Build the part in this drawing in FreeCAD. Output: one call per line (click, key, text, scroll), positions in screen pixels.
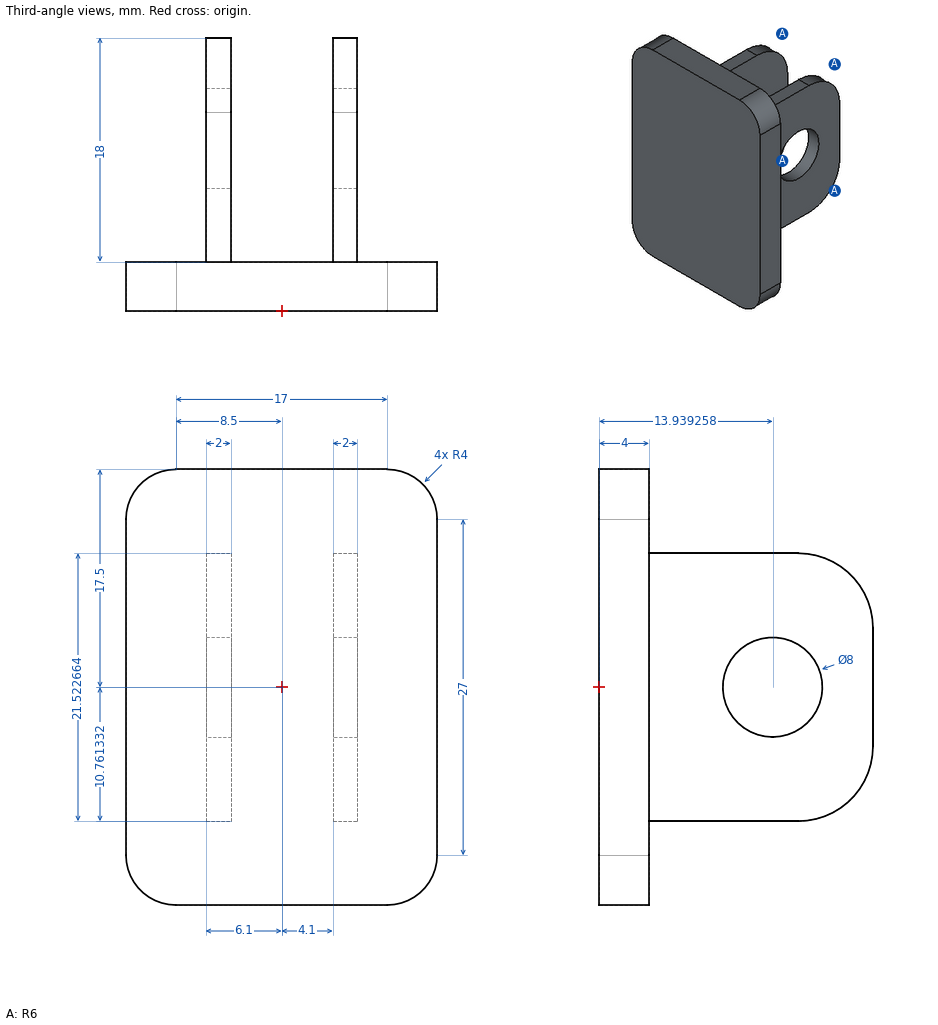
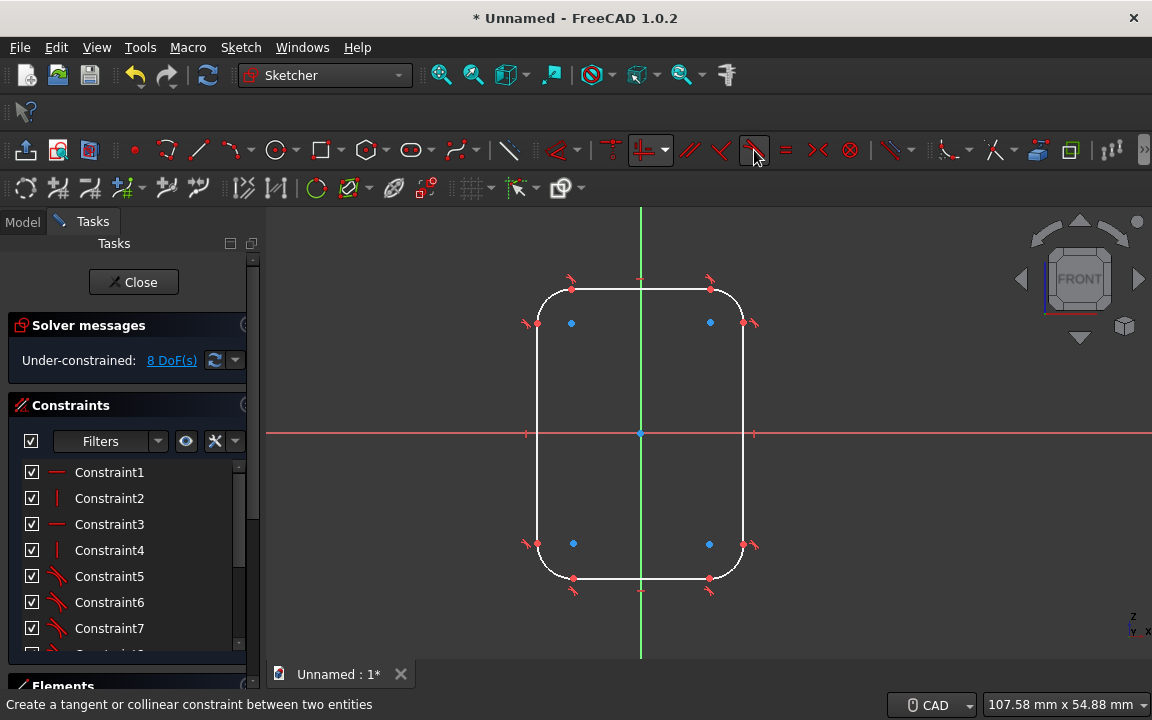
click(740, 307)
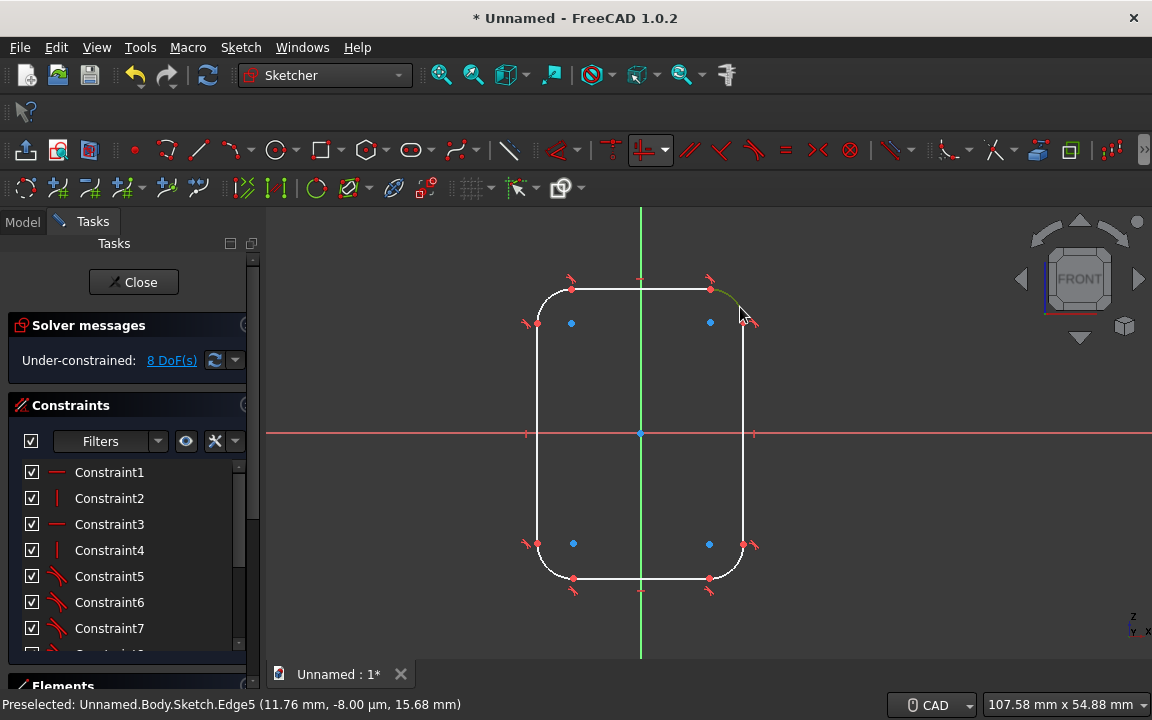
click(725, 575)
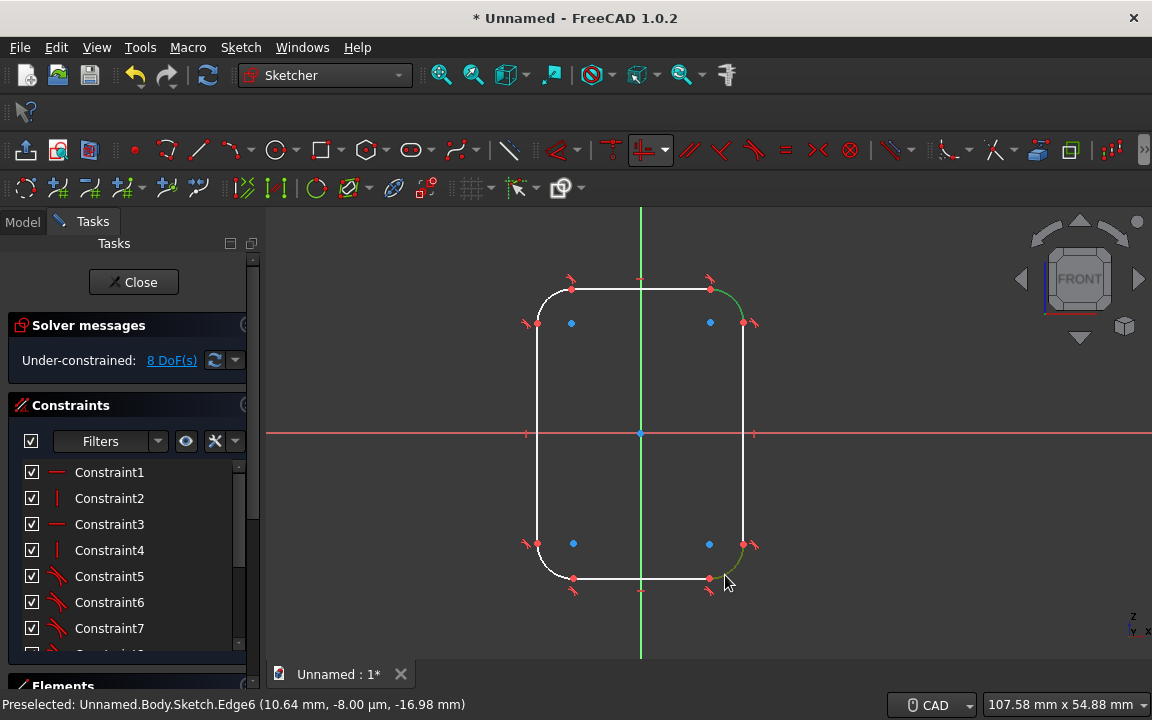
click(541, 559)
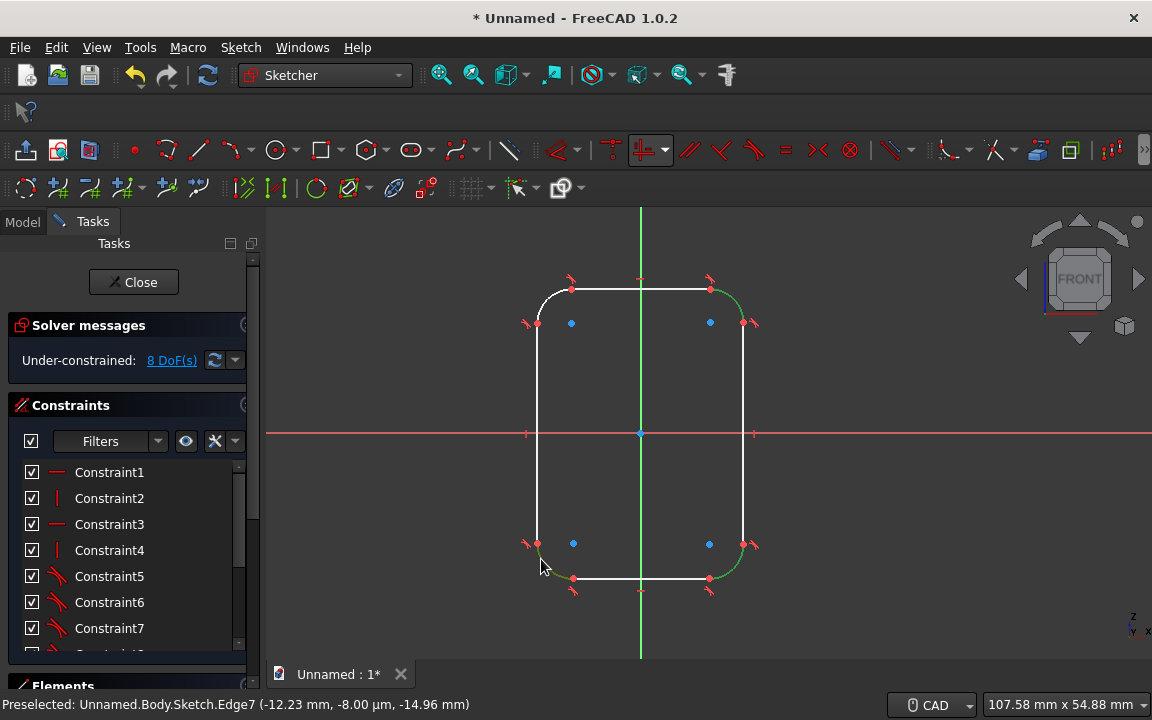
click(556, 293)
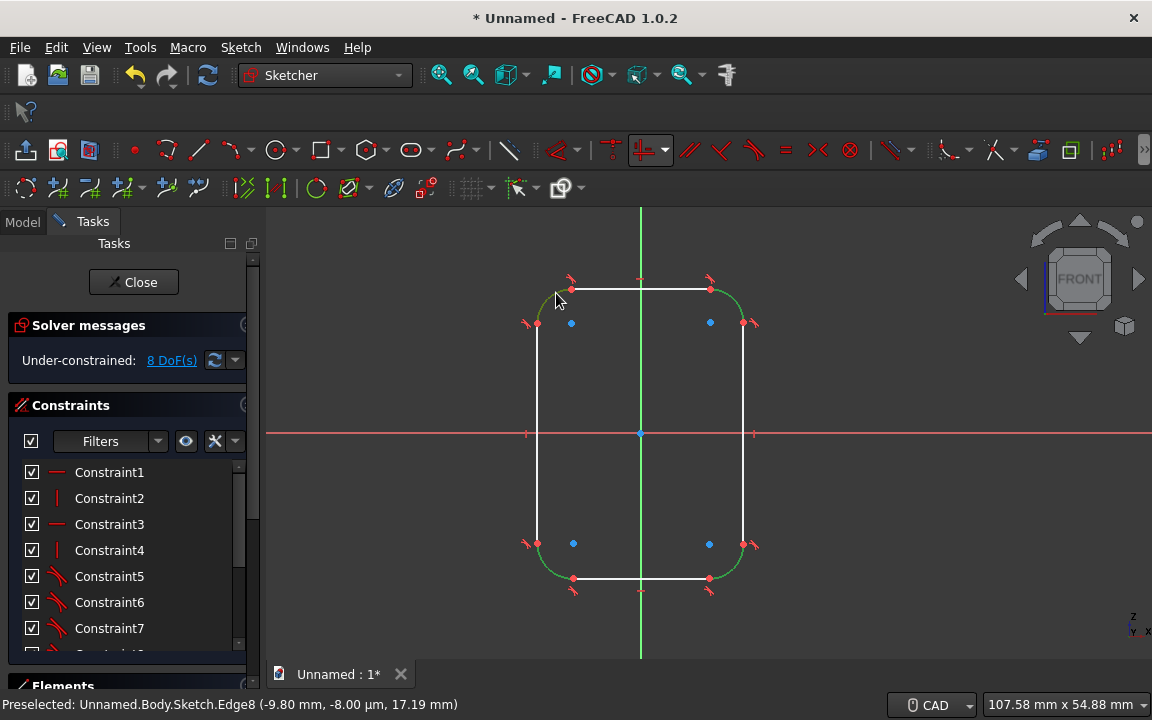
click(786, 150)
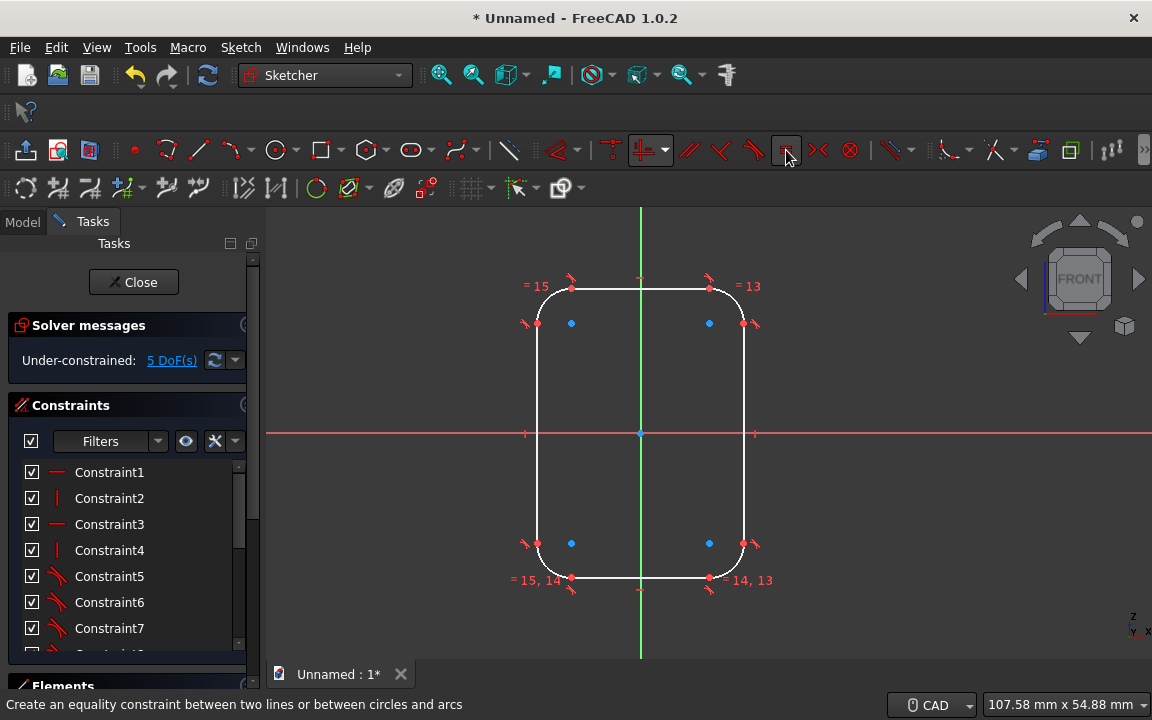
click(556, 150)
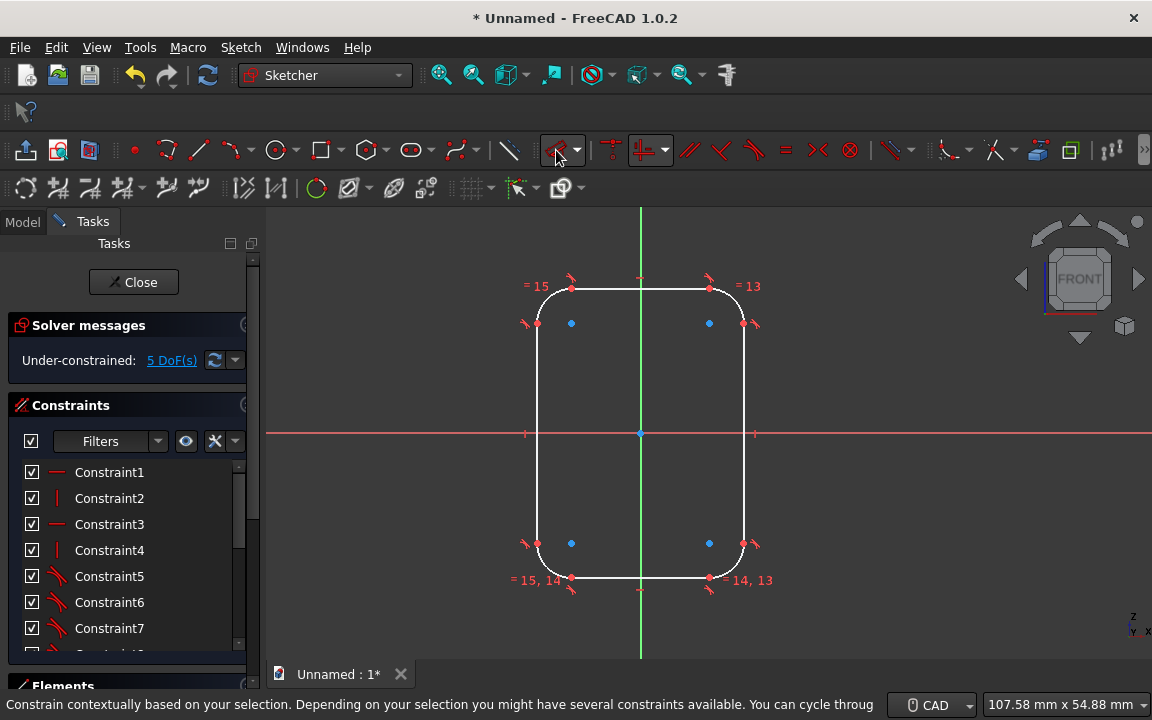
click(740, 308)
click(769, 293)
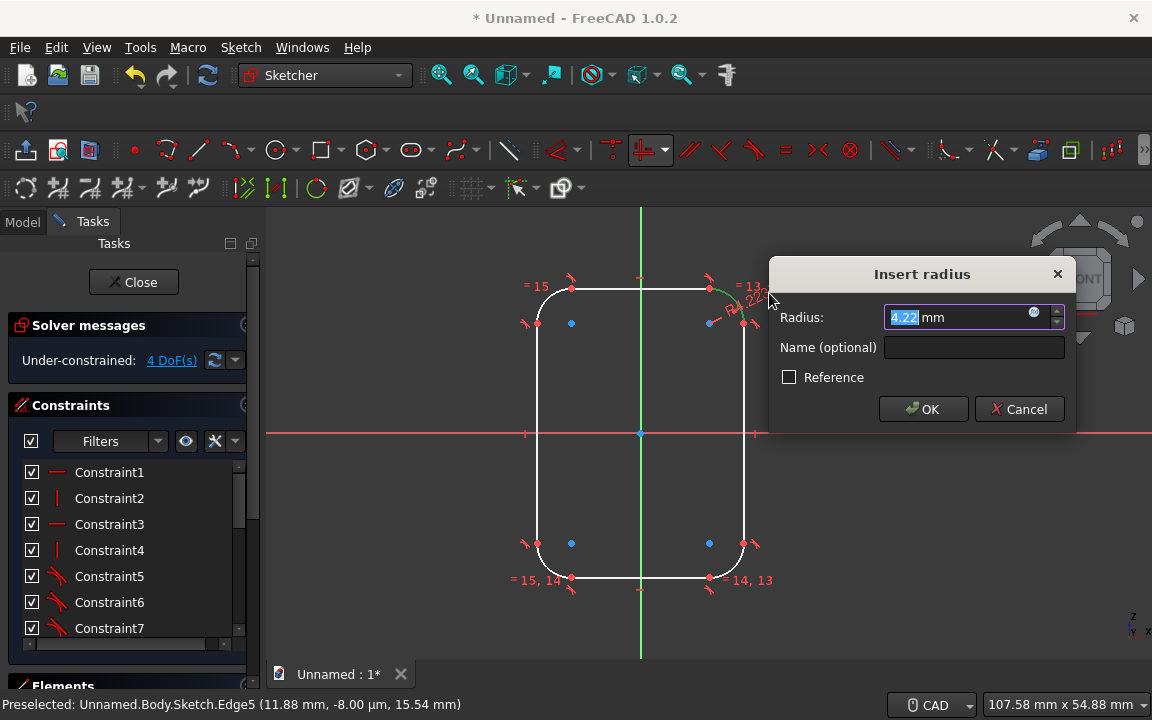
text(4)
key(Return)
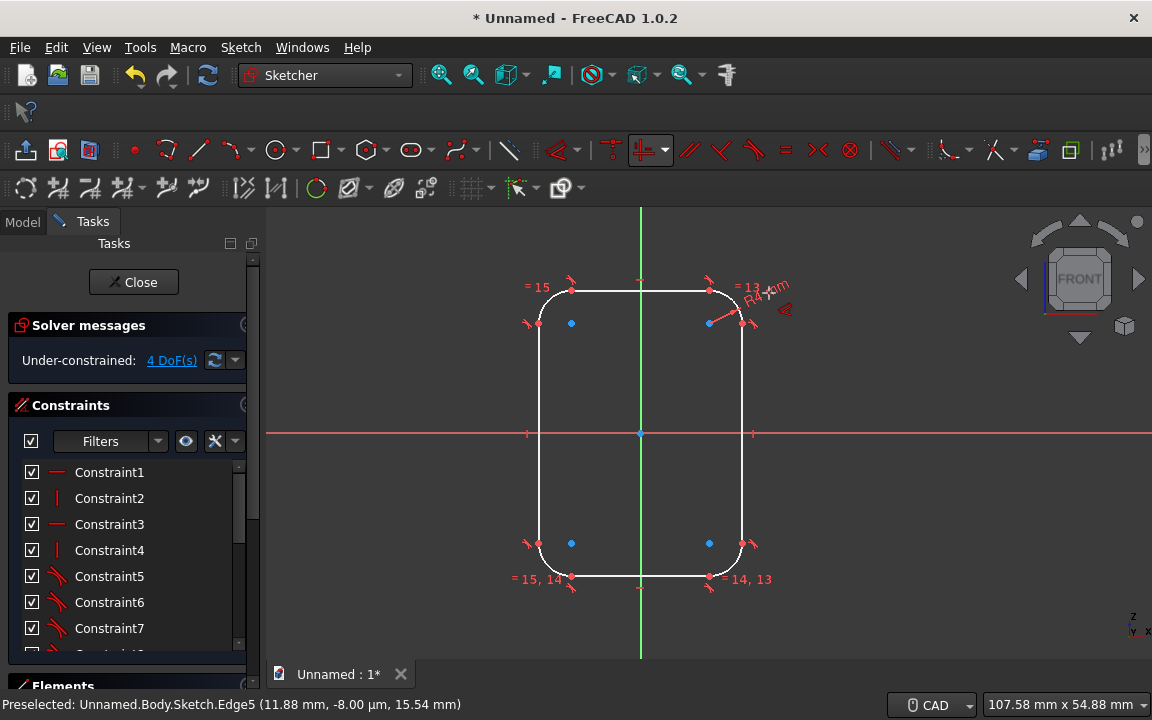
click(613, 291)
click(609, 257)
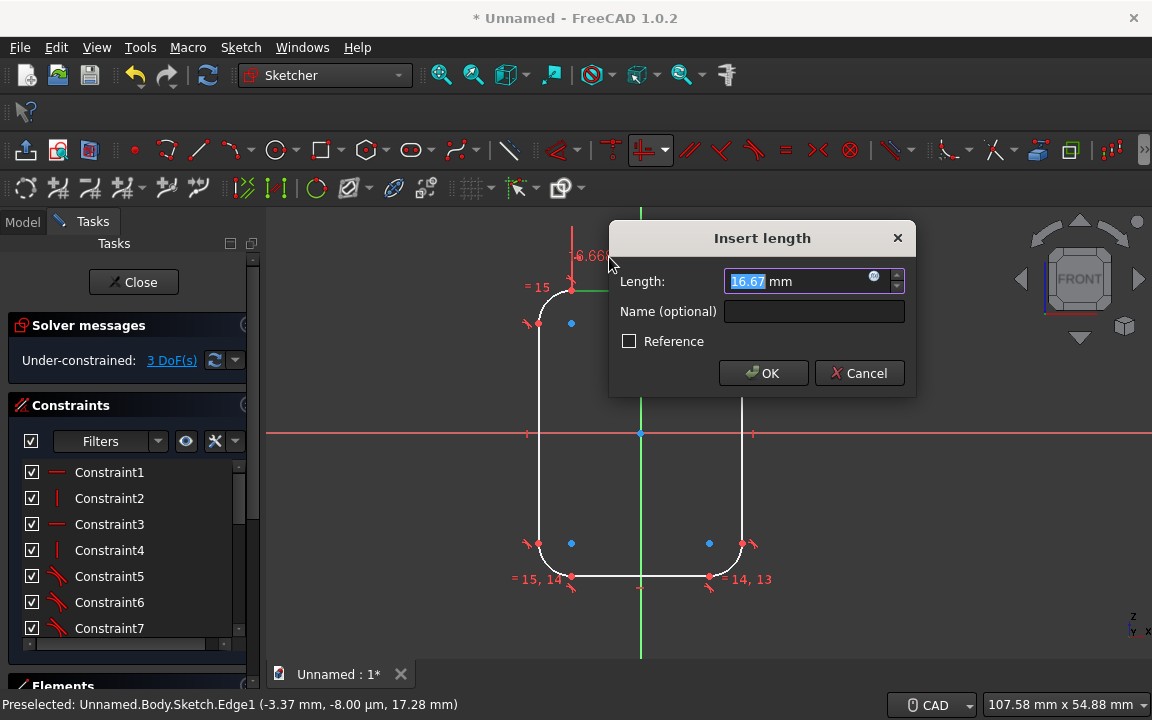
text(17)
key(Return)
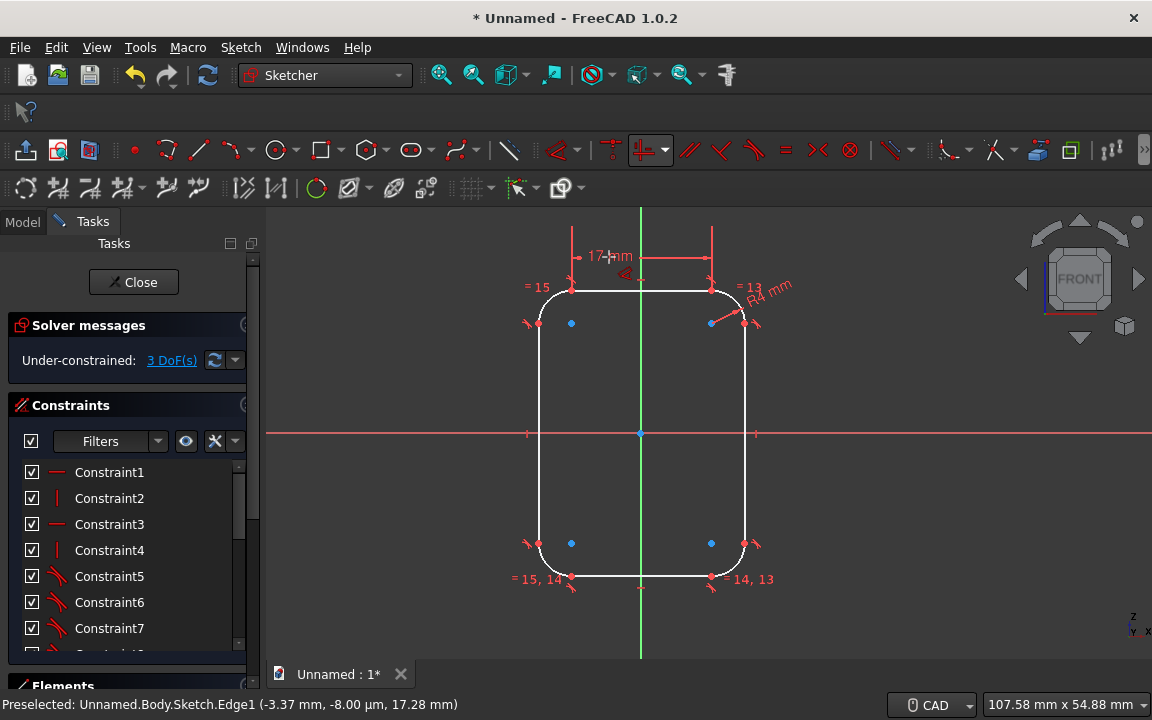
click(745, 390)
click(779, 383)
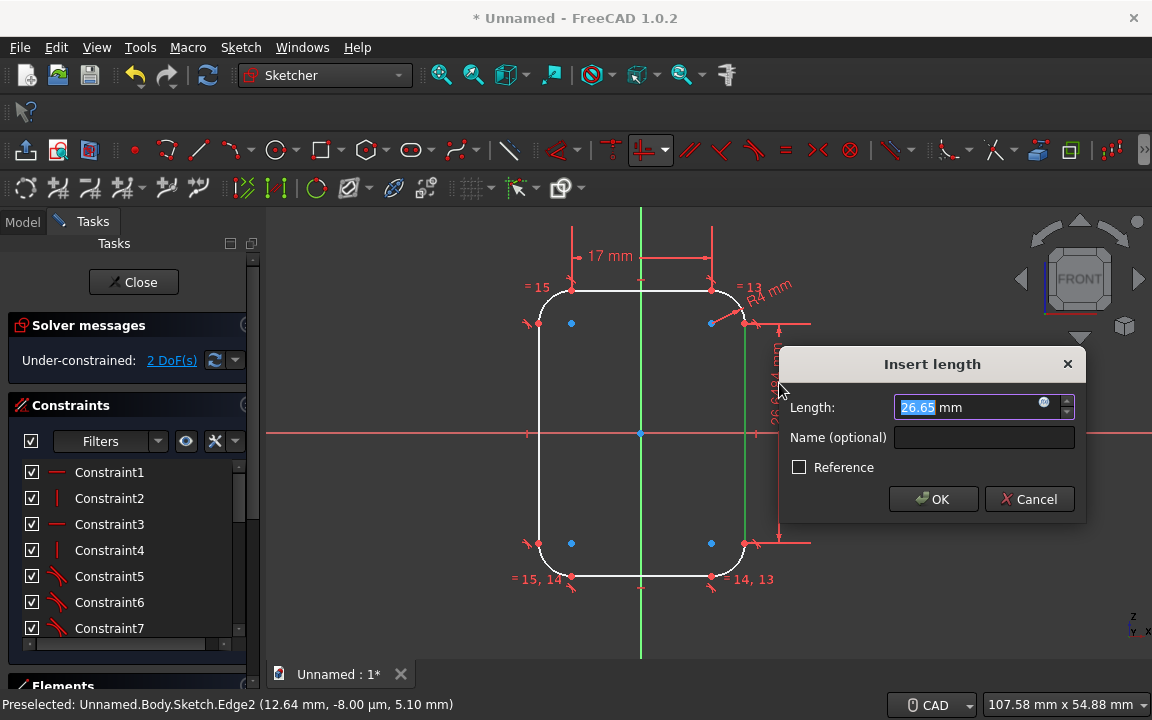
text(27)
key(Return)